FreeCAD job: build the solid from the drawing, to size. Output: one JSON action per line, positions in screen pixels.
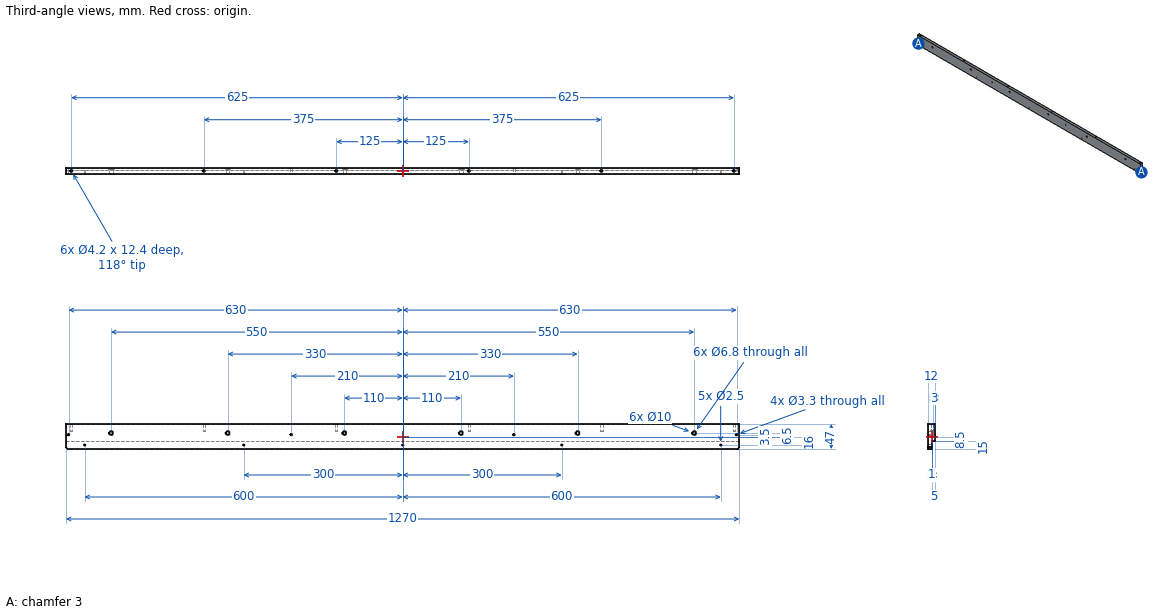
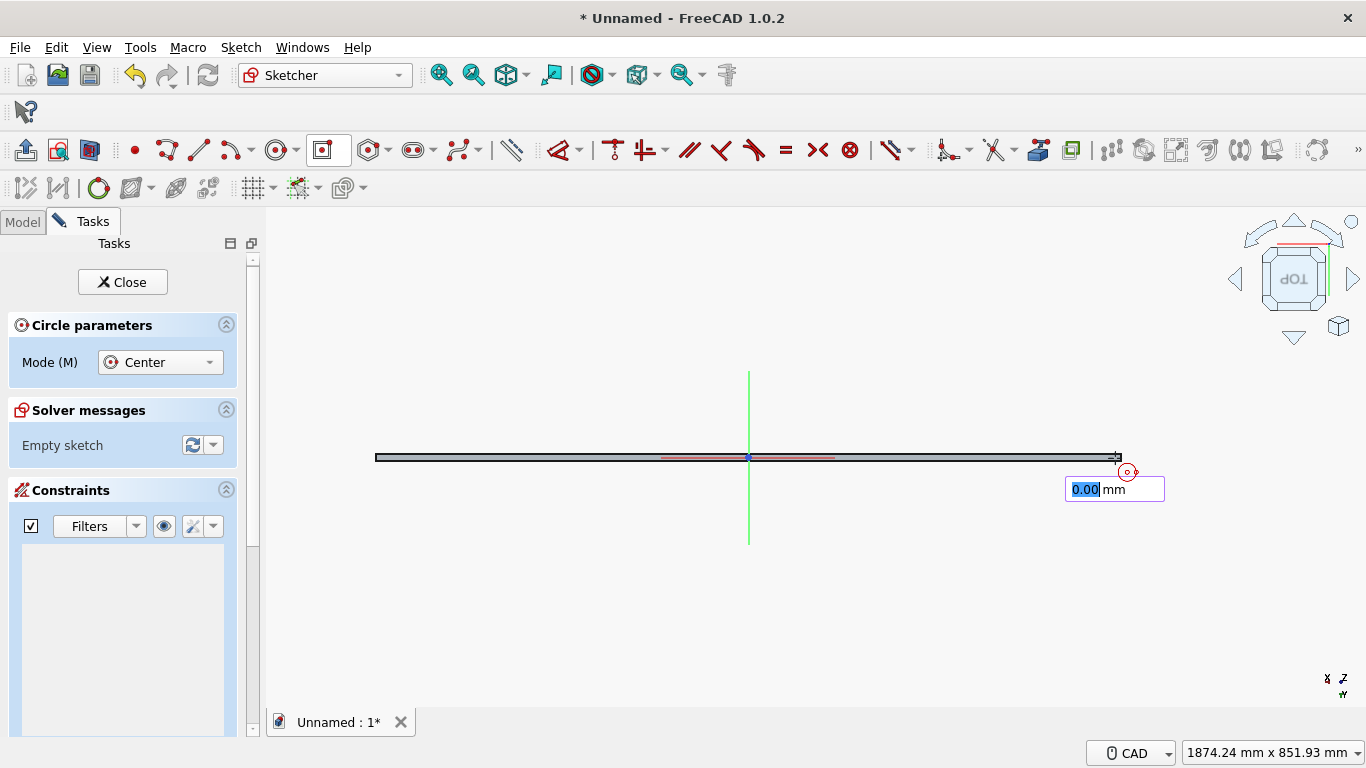
{"action": "scroll", "coordinate": [1116, 456], "scroll_direction": "up", "scroll_amount": 14}
{"action": "mouse_move", "coordinate": [1101, 456]}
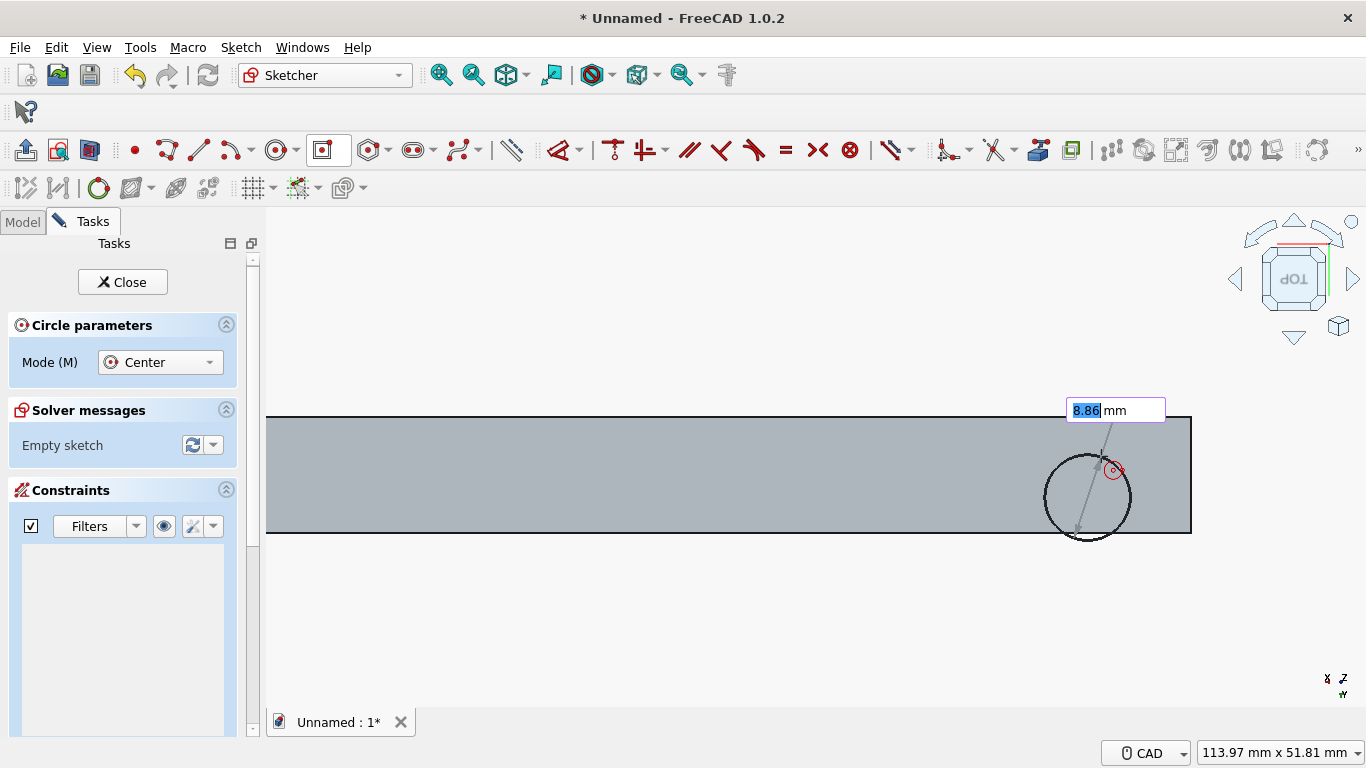
{"action": "type", "text": "4.2"}
{"action": "key", "text": "Return"}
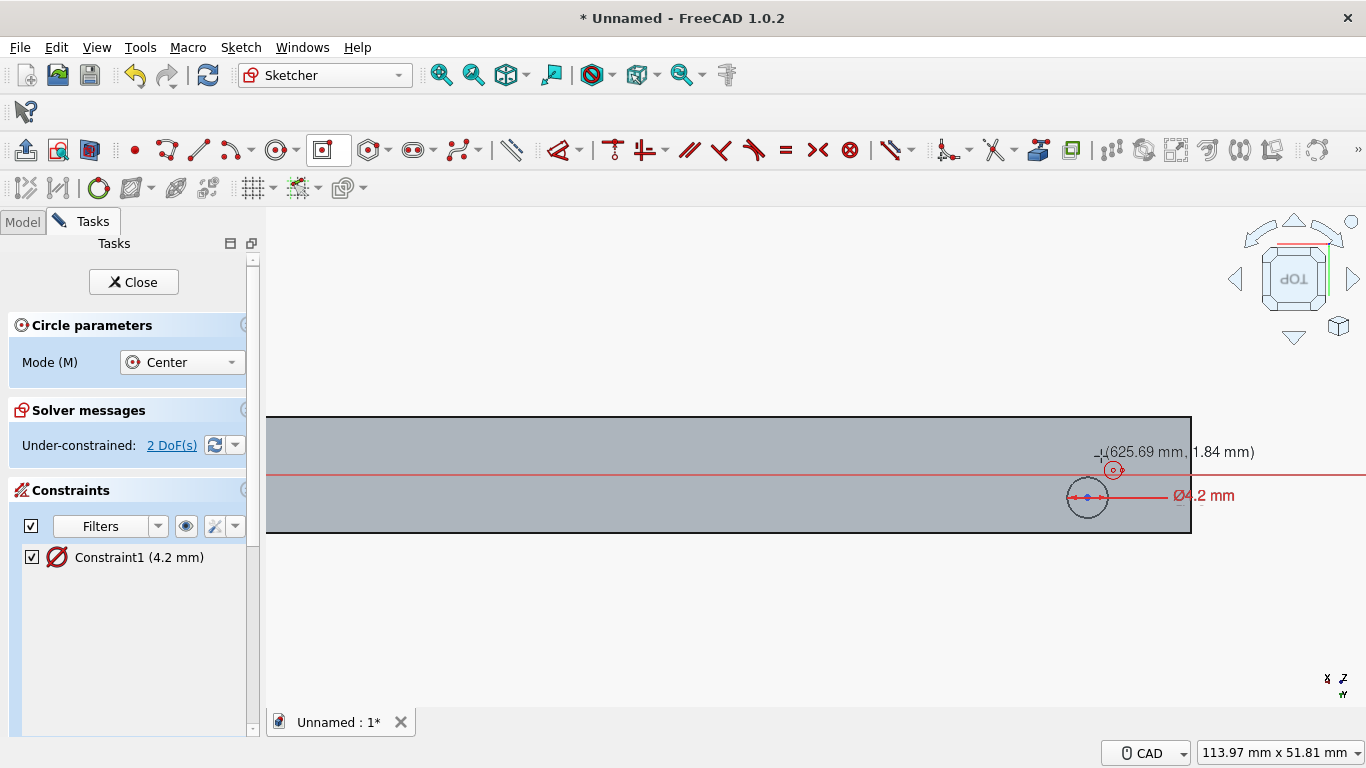
{"action": "scroll", "coordinate": [1045, 456], "scroll_direction": "down", "scroll_amount": 15}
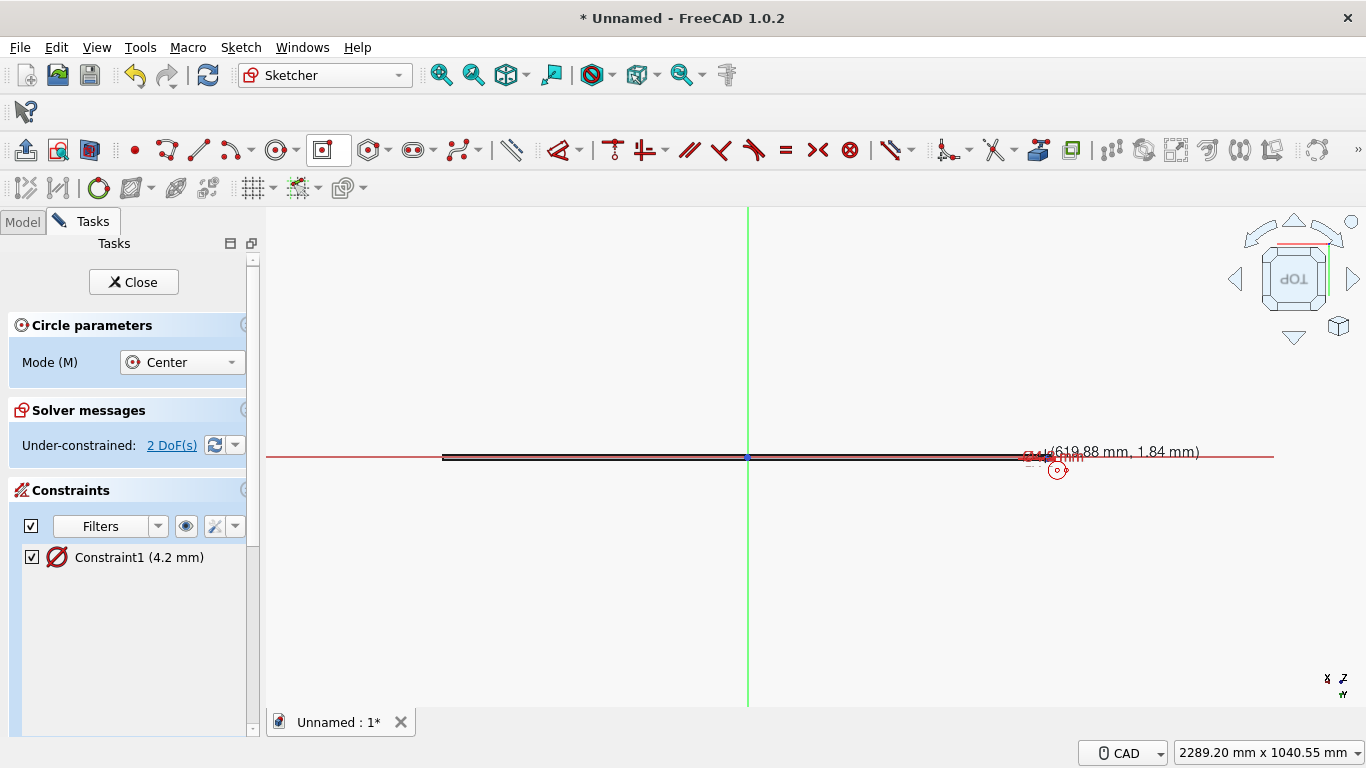
{"action": "scroll", "coordinate": [928, 457], "scroll_direction": "up", "scroll_amount": 16}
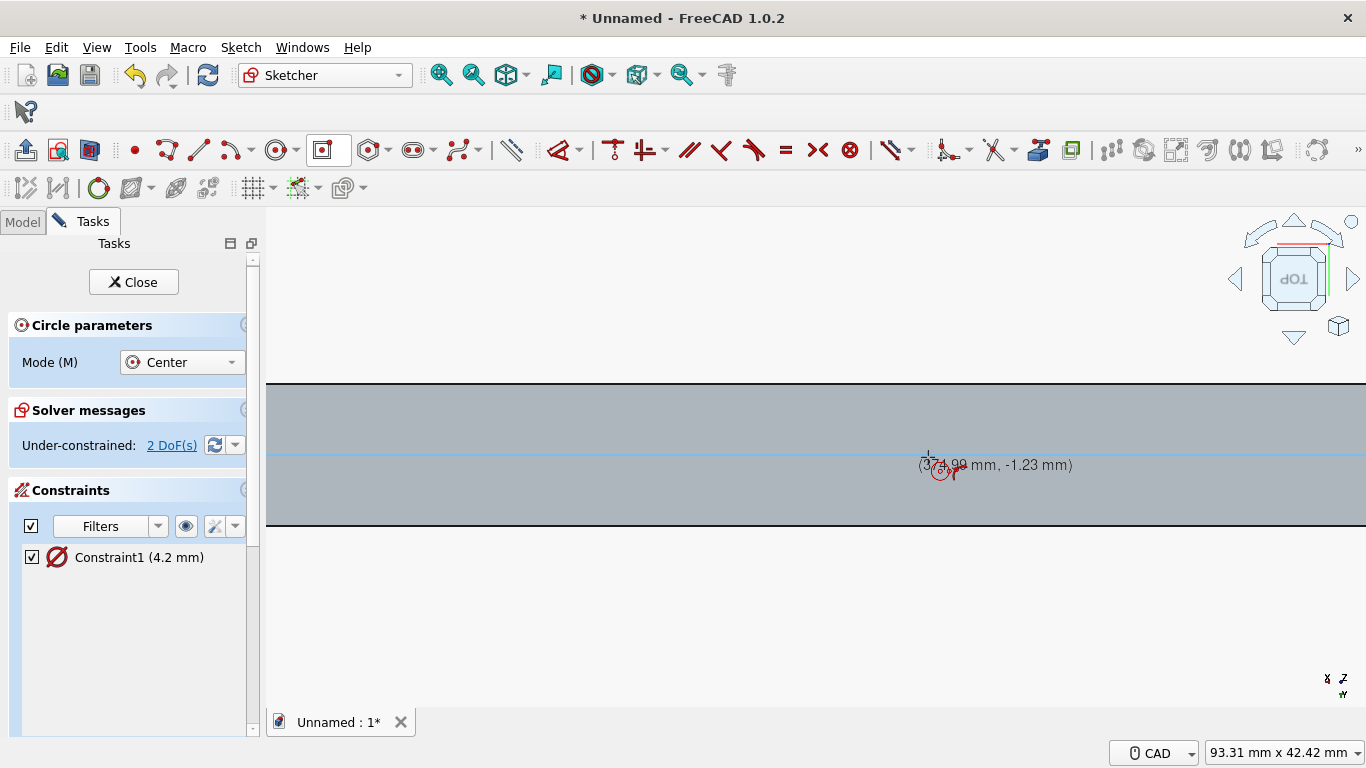
{"action": "scroll", "coordinate": [970, 457], "scroll_direction": "down", "scroll_amount": 15}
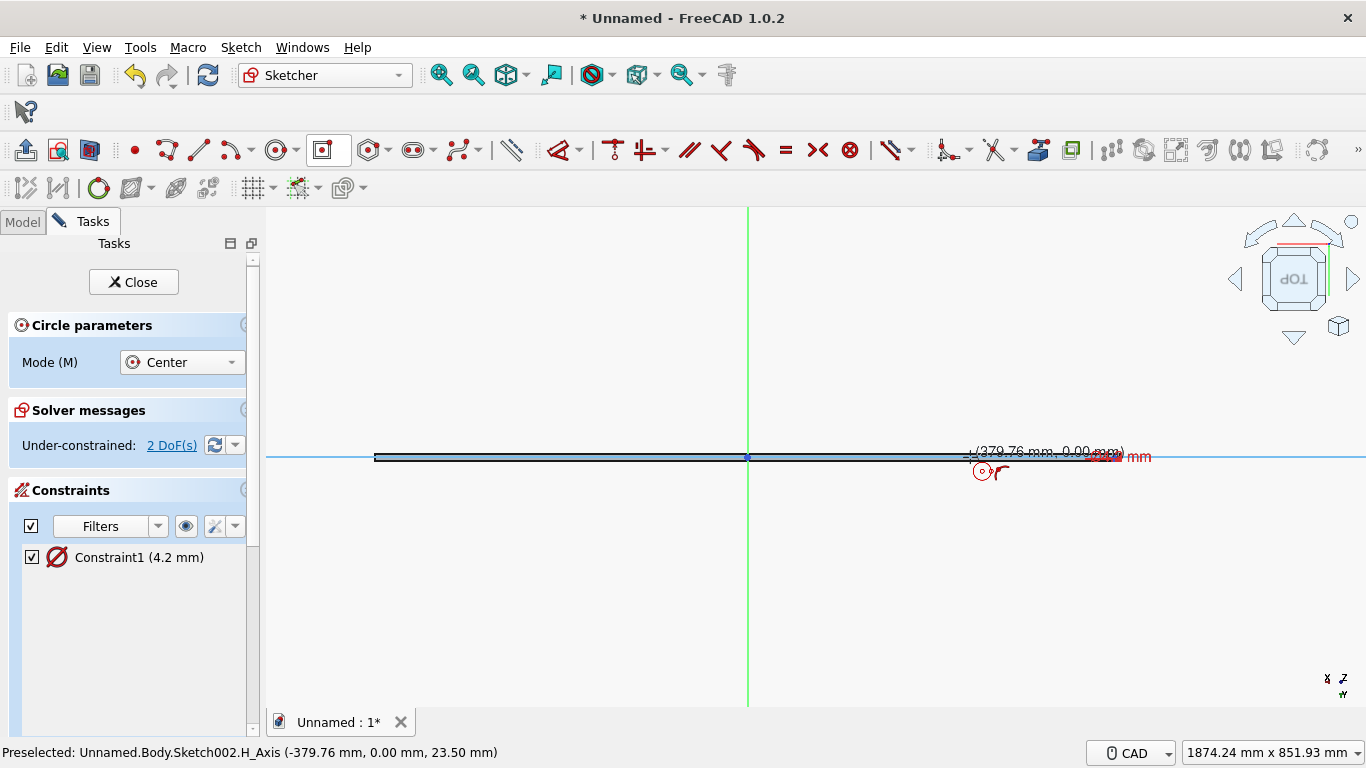
{"action": "left_click", "coordinate": [968, 457]}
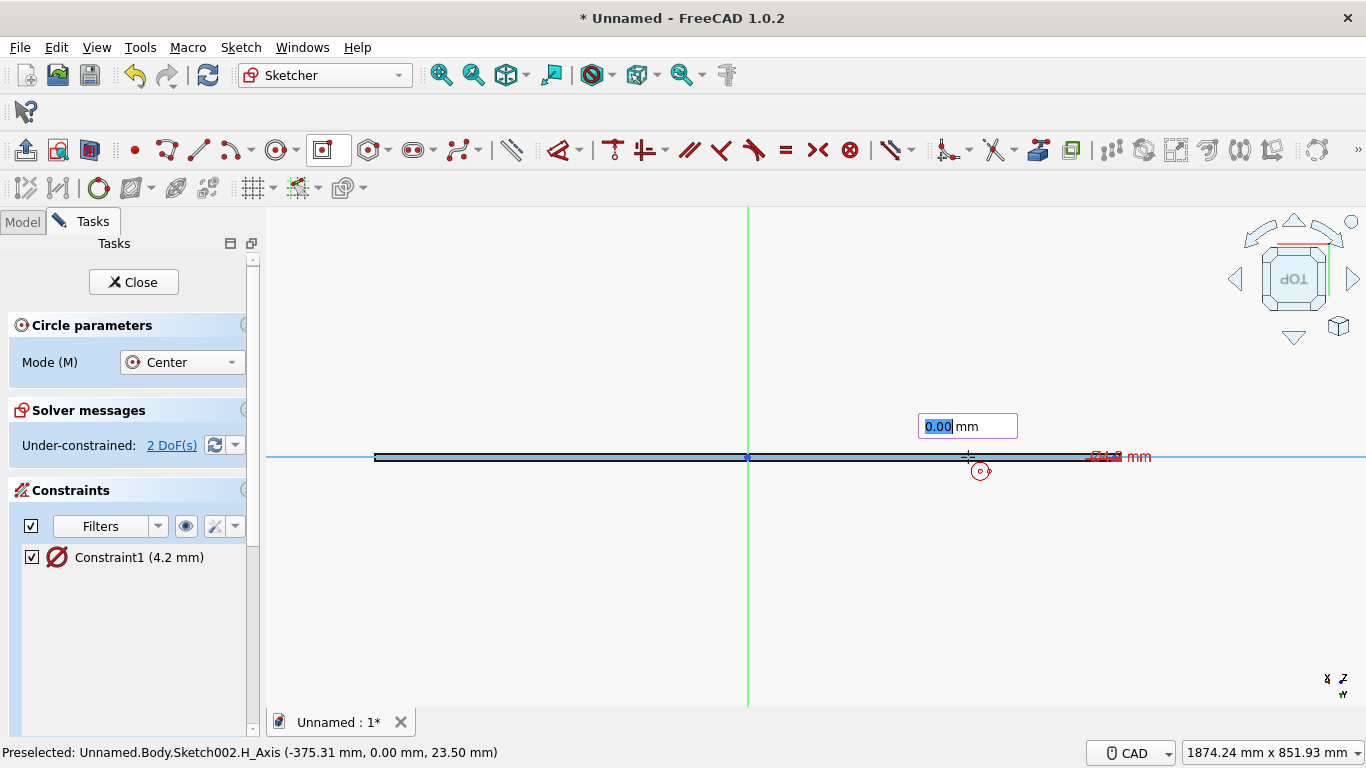
{"action": "scroll", "coordinate": [968, 456], "scroll_direction": "up", "scroll_amount": 14}
{"action": "mouse_move", "coordinate": [962, 452]}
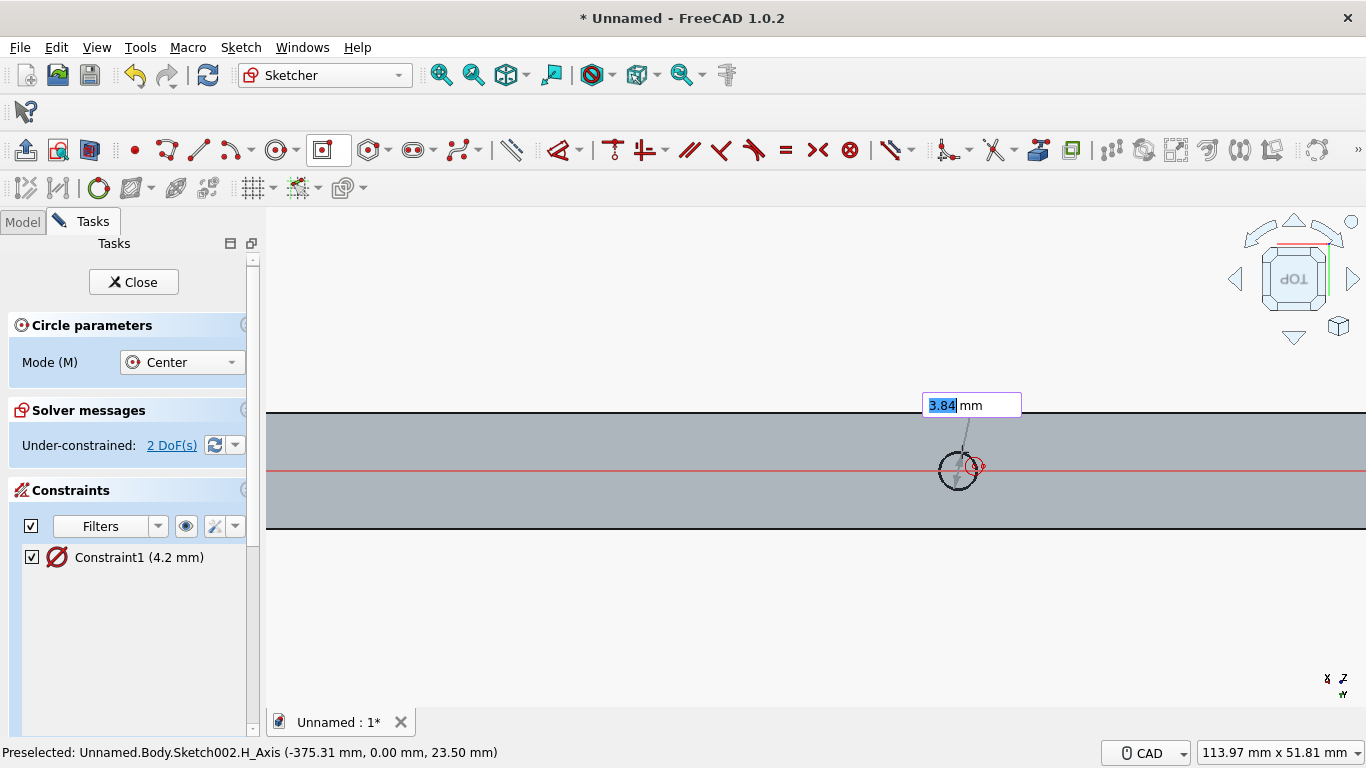
{"action": "type", "text": "4.2"}
{"action": "key", "text": "Return"}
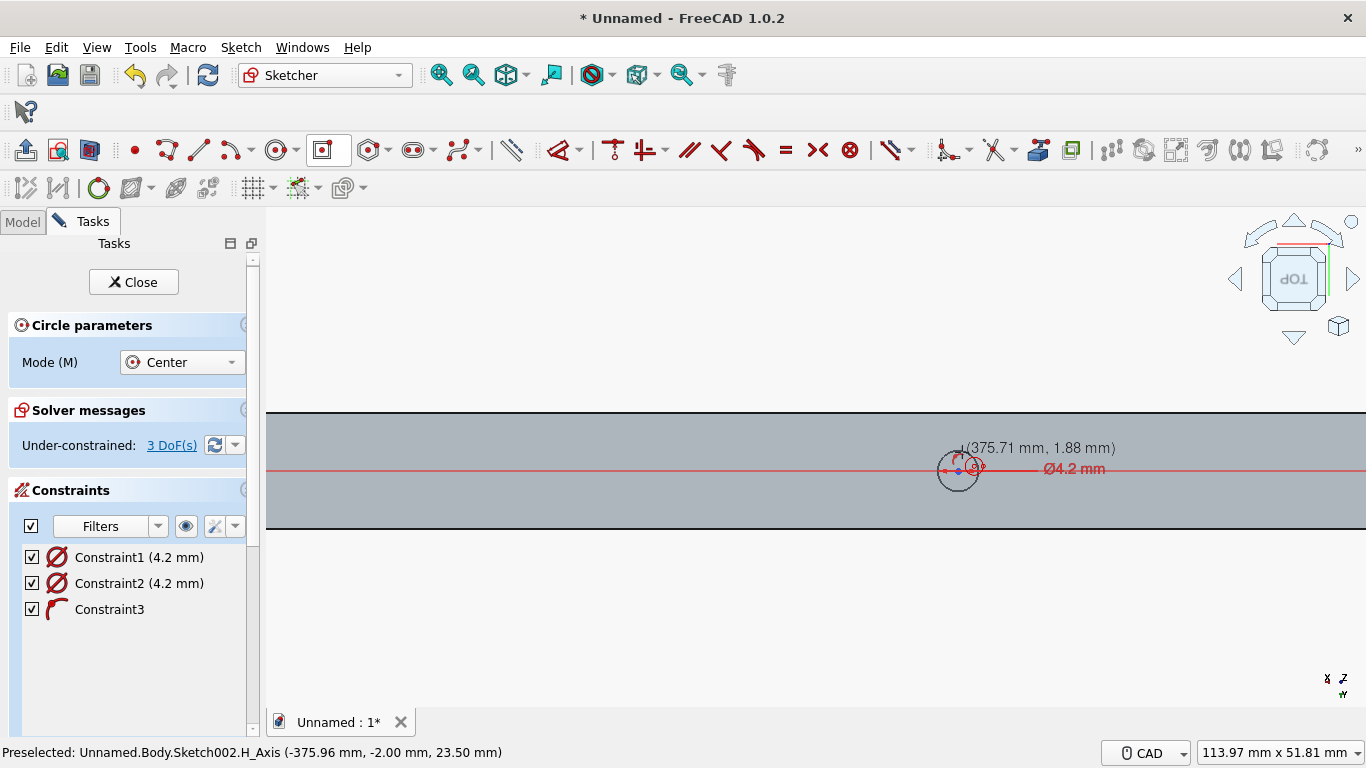
{"action": "scroll", "coordinate": [926, 456], "scroll_direction": "down", "scroll_amount": 15}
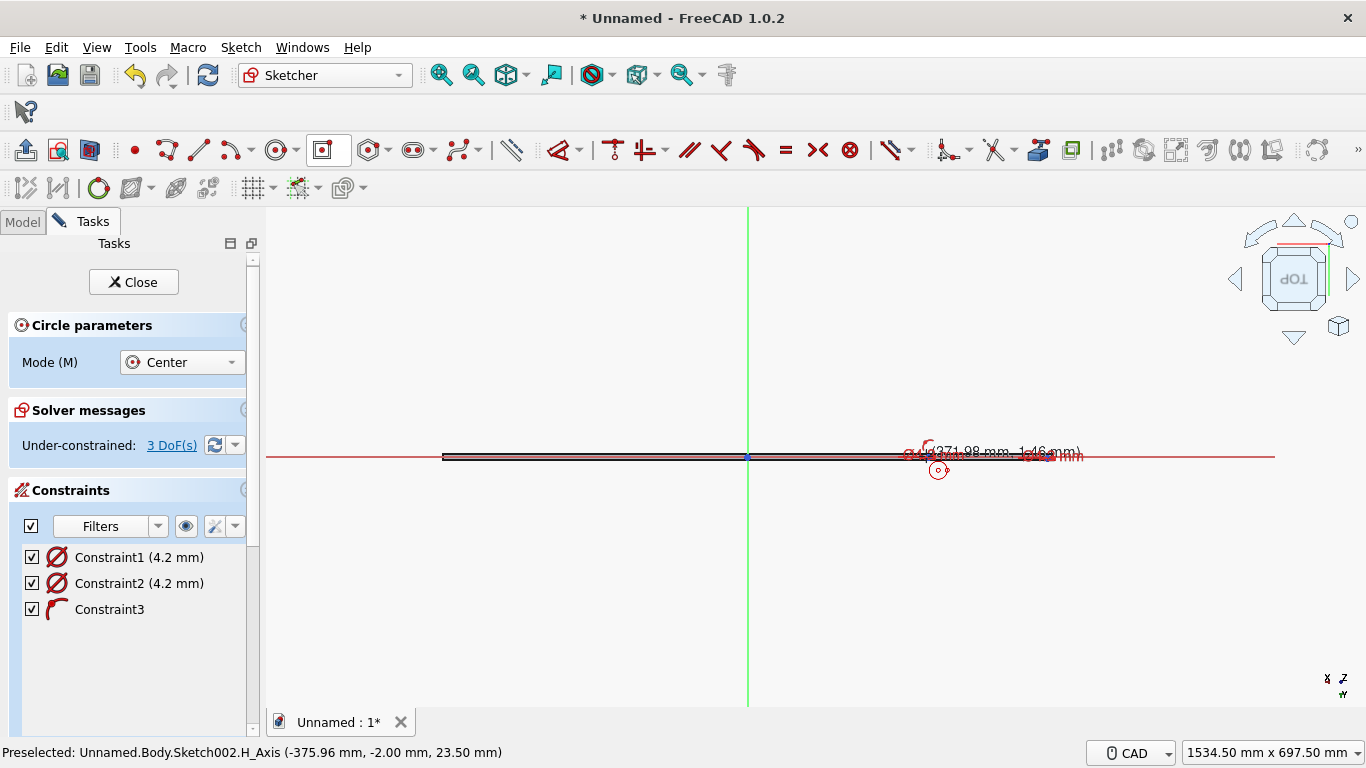
{"action": "scroll", "coordinate": [808, 457], "scroll_direction": "up", "scroll_amount": 16}